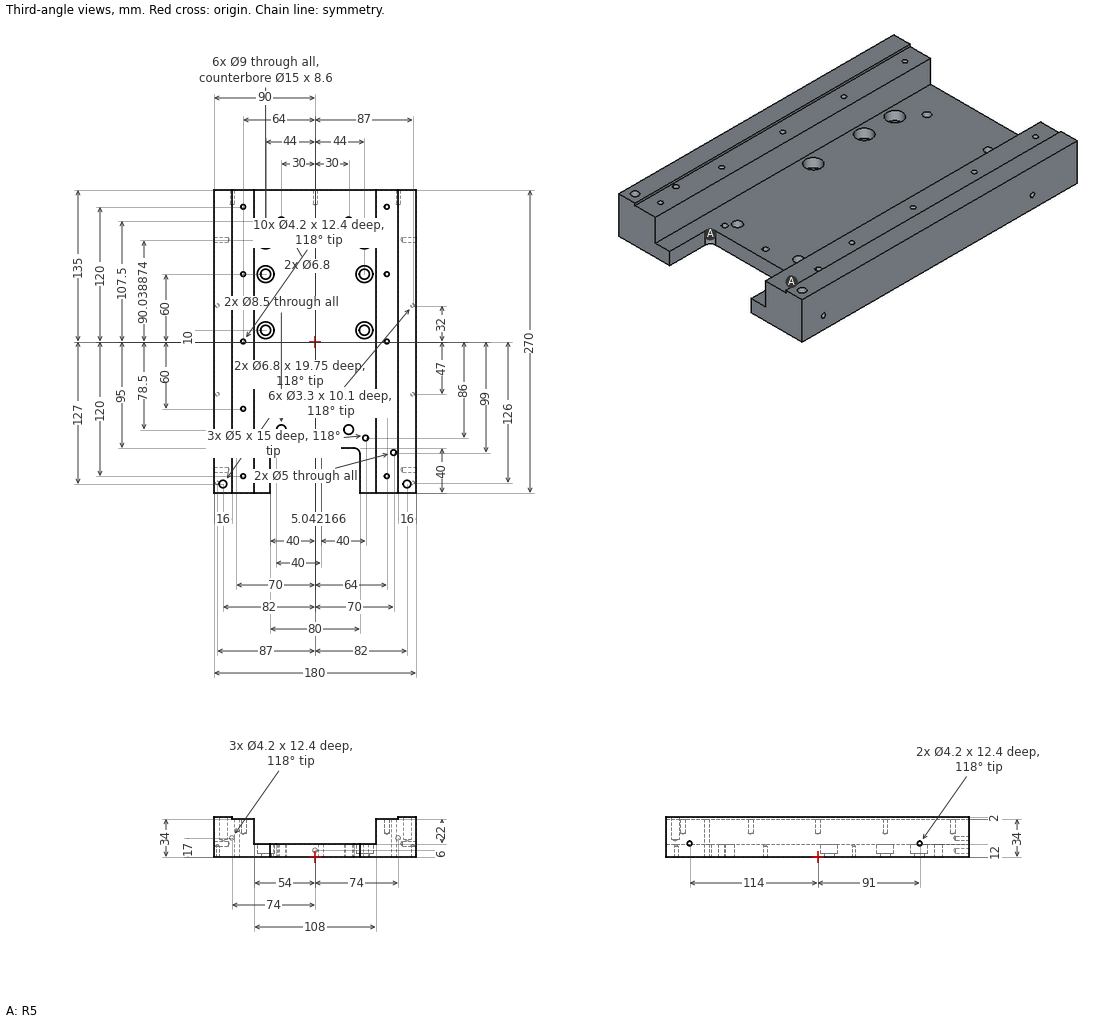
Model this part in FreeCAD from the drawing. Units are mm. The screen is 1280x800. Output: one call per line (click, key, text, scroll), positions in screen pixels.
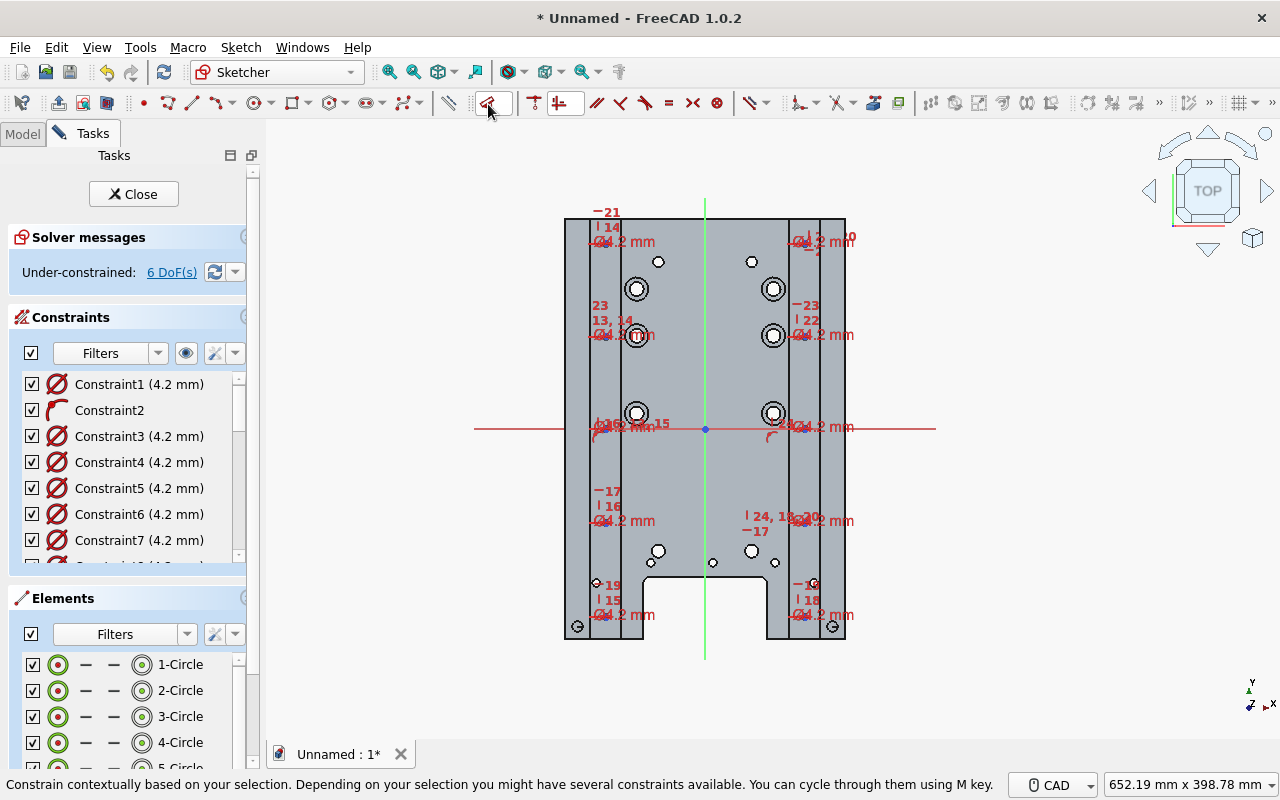
click(606, 429)
click(656, 463)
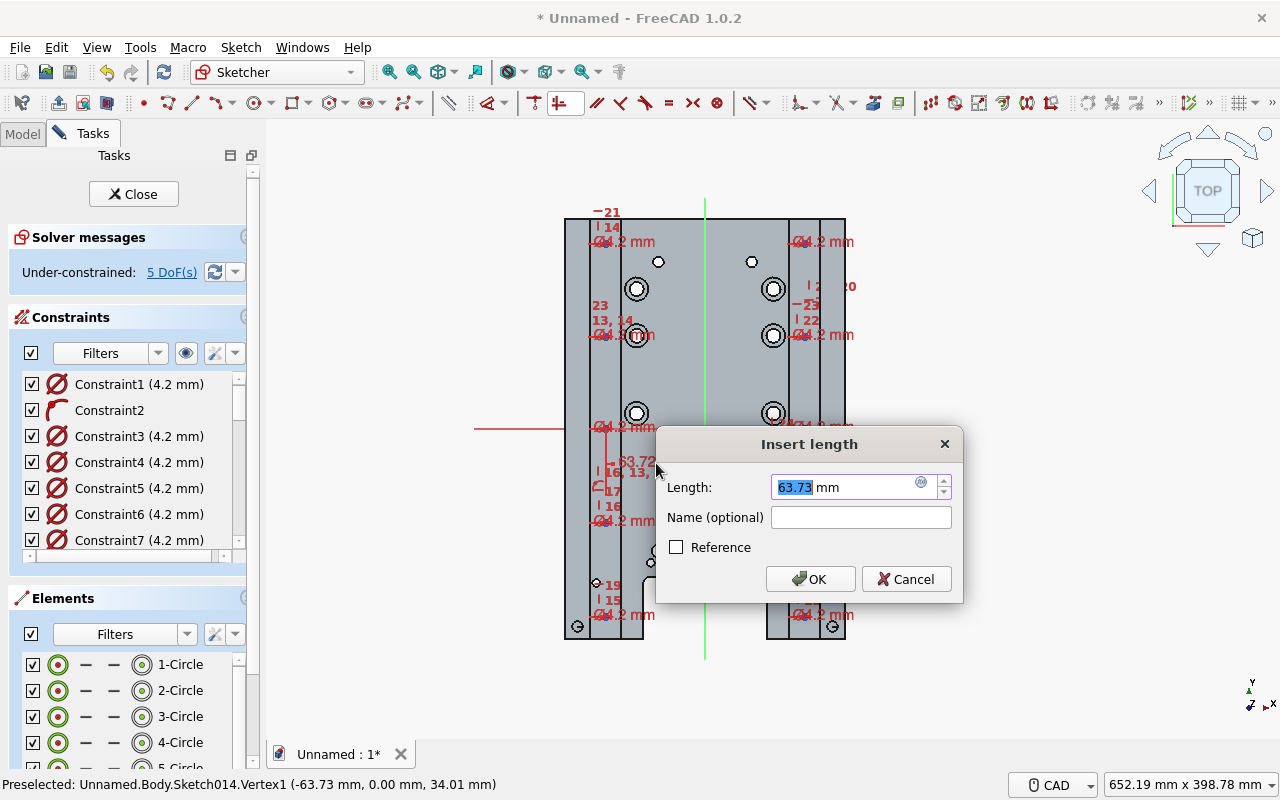
text(64)
key(Return)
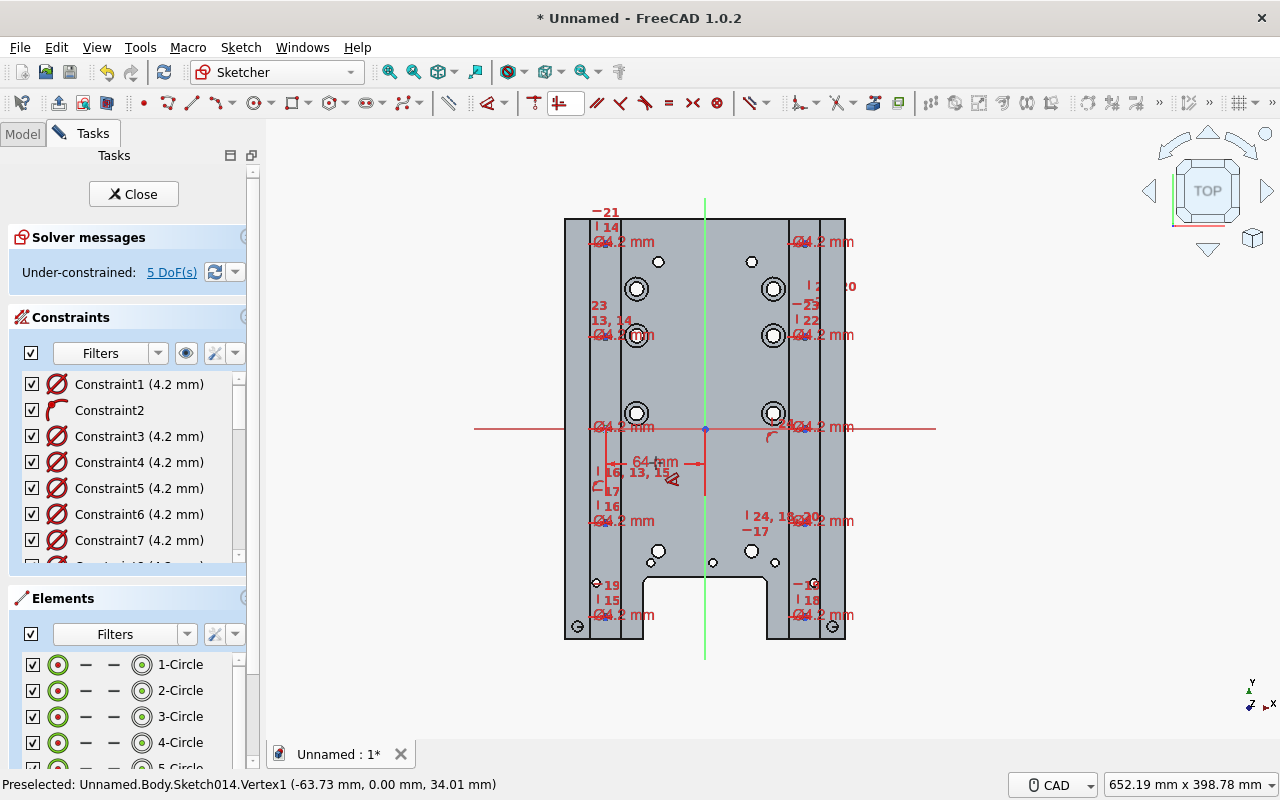
click(606, 337)
click(572, 383)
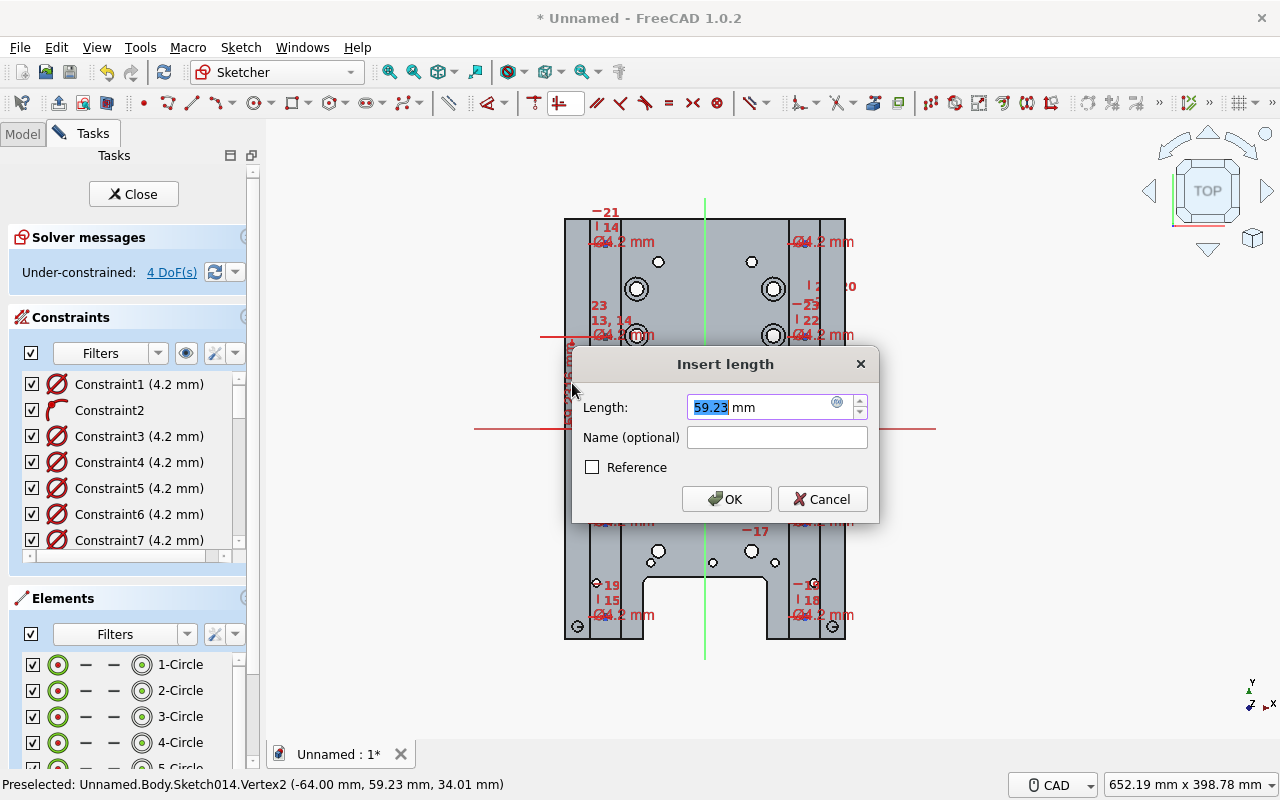
text(60)
key(Return)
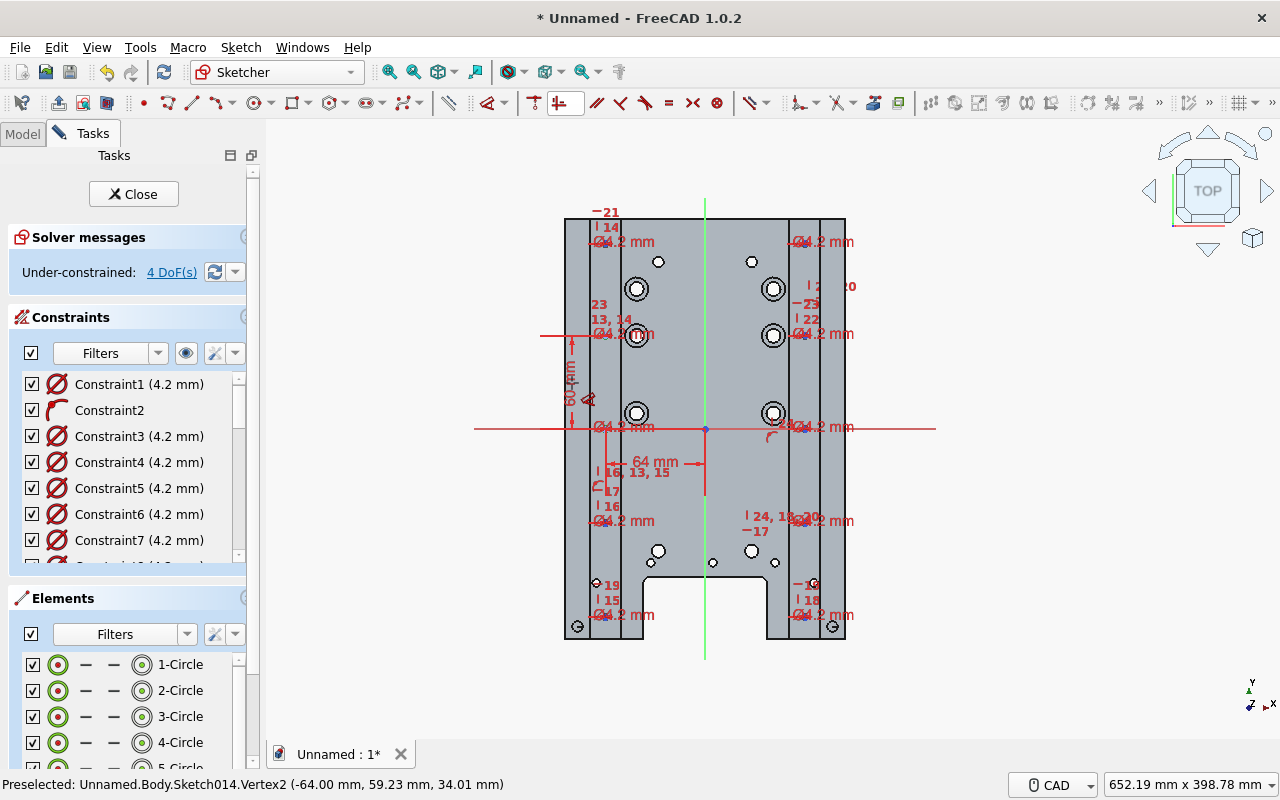
click(606, 523)
click(572, 476)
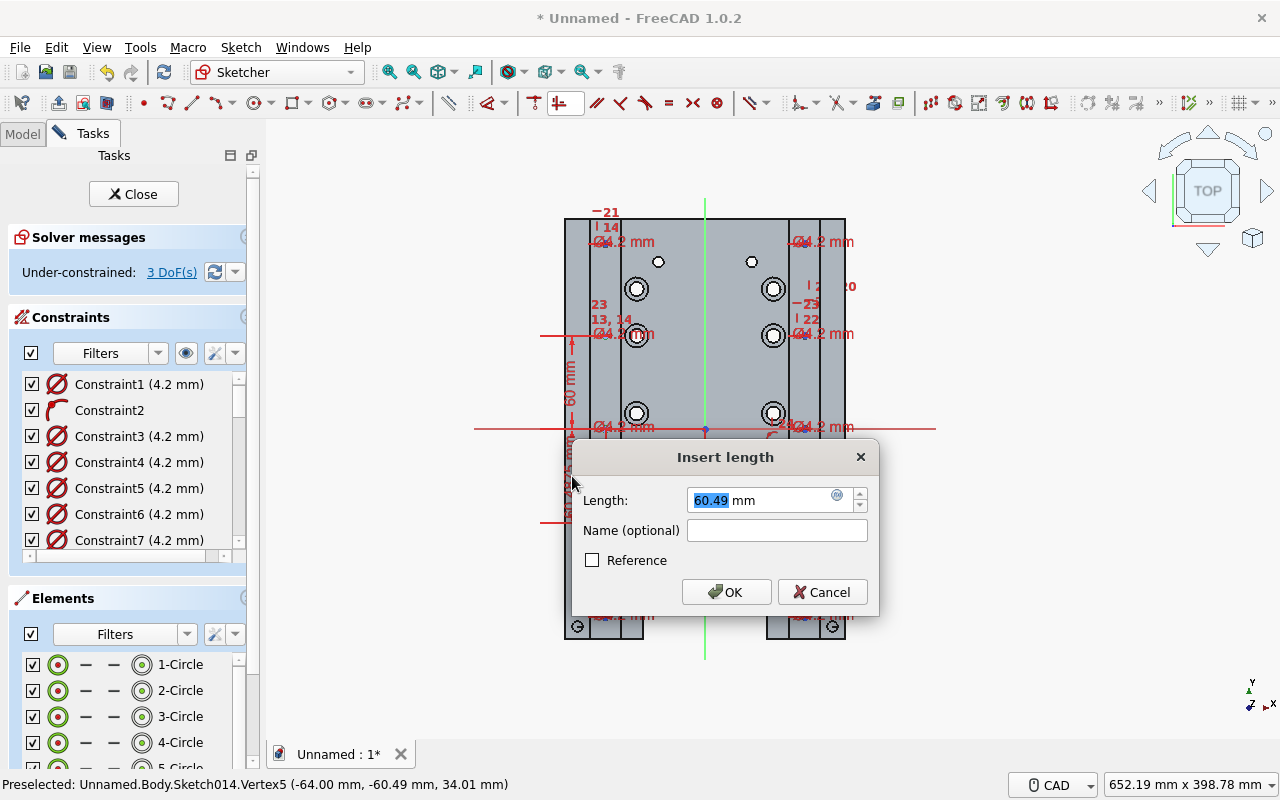
text(60)
key(Return)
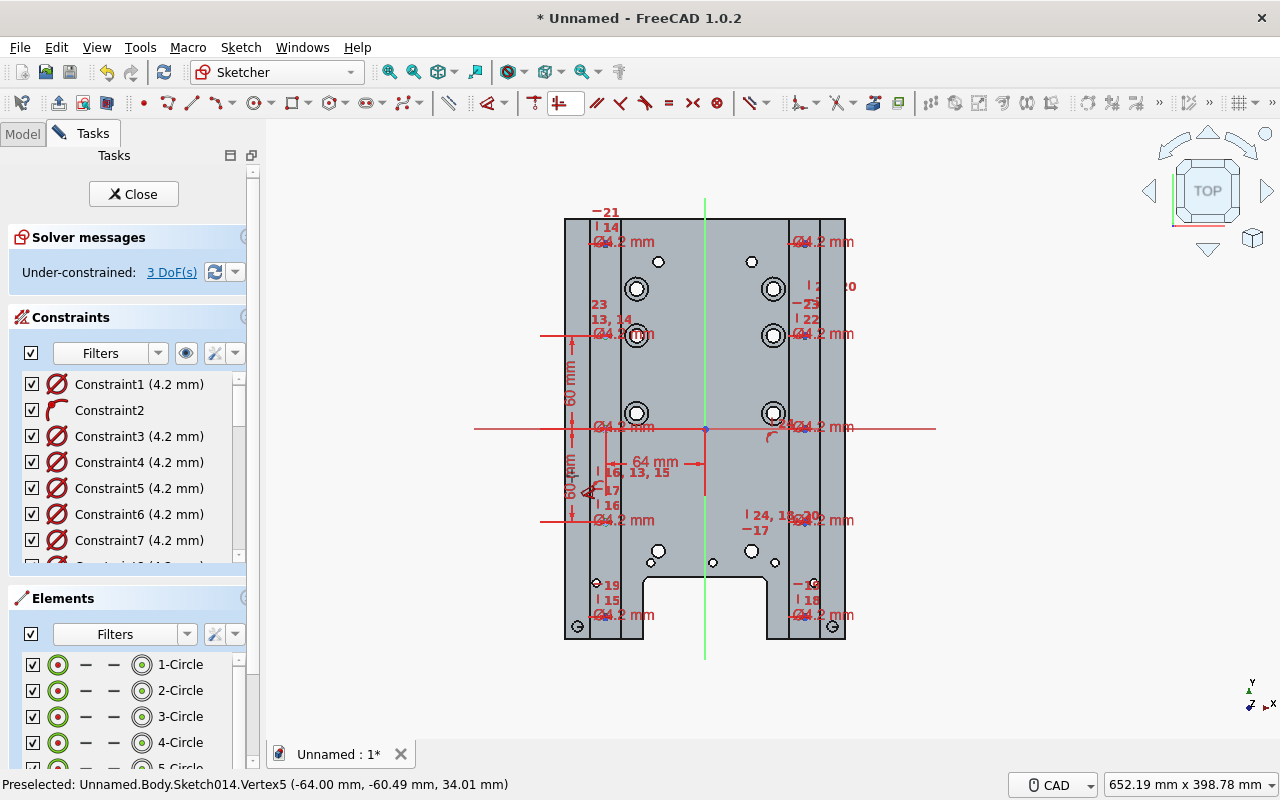
click(805, 522)
click(755, 556)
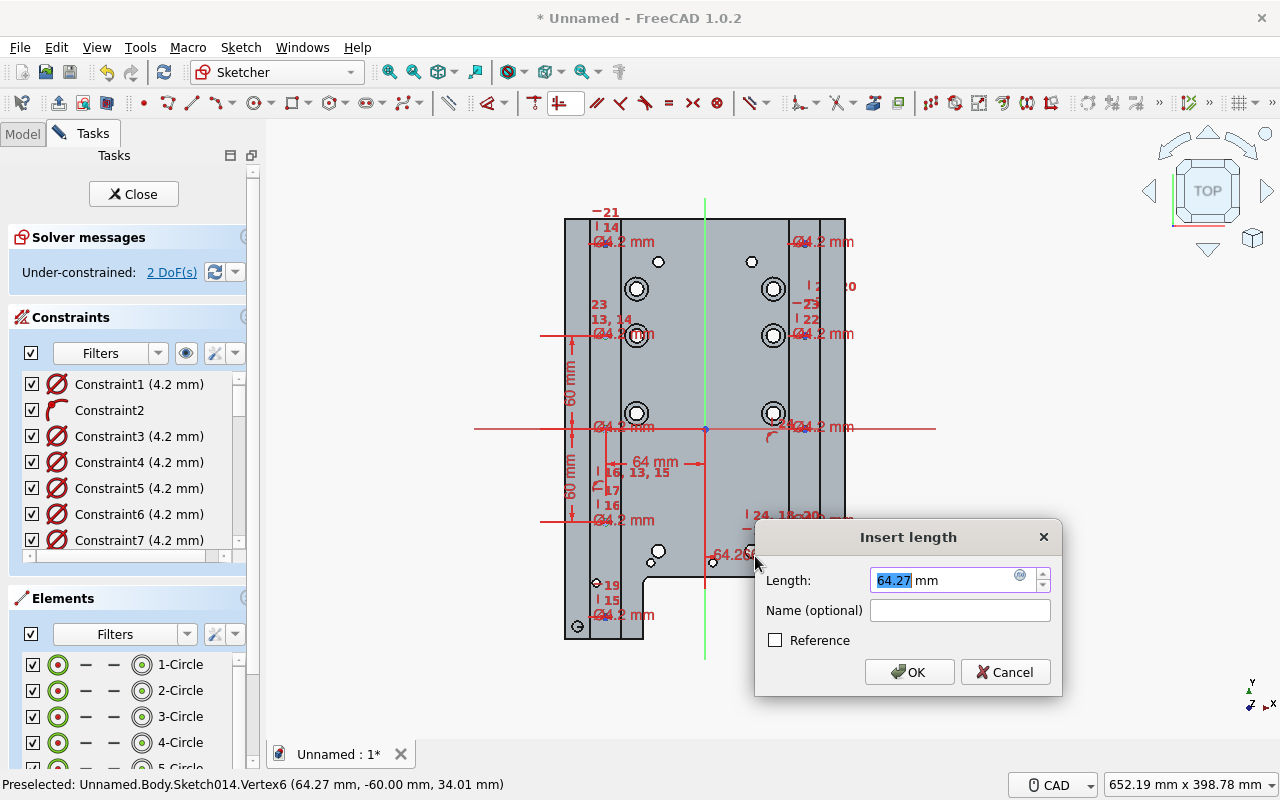
text(64)
key(Return)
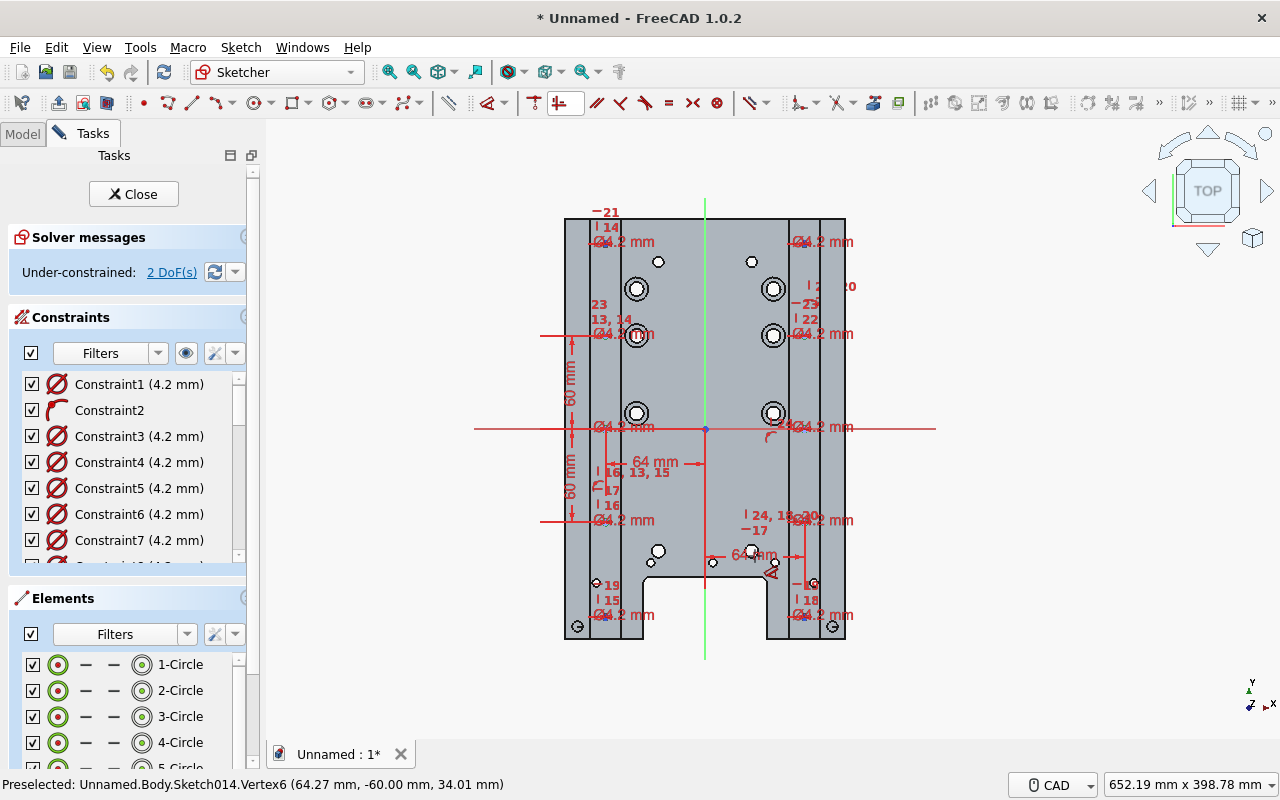
click(606, 244)
click(572, 337)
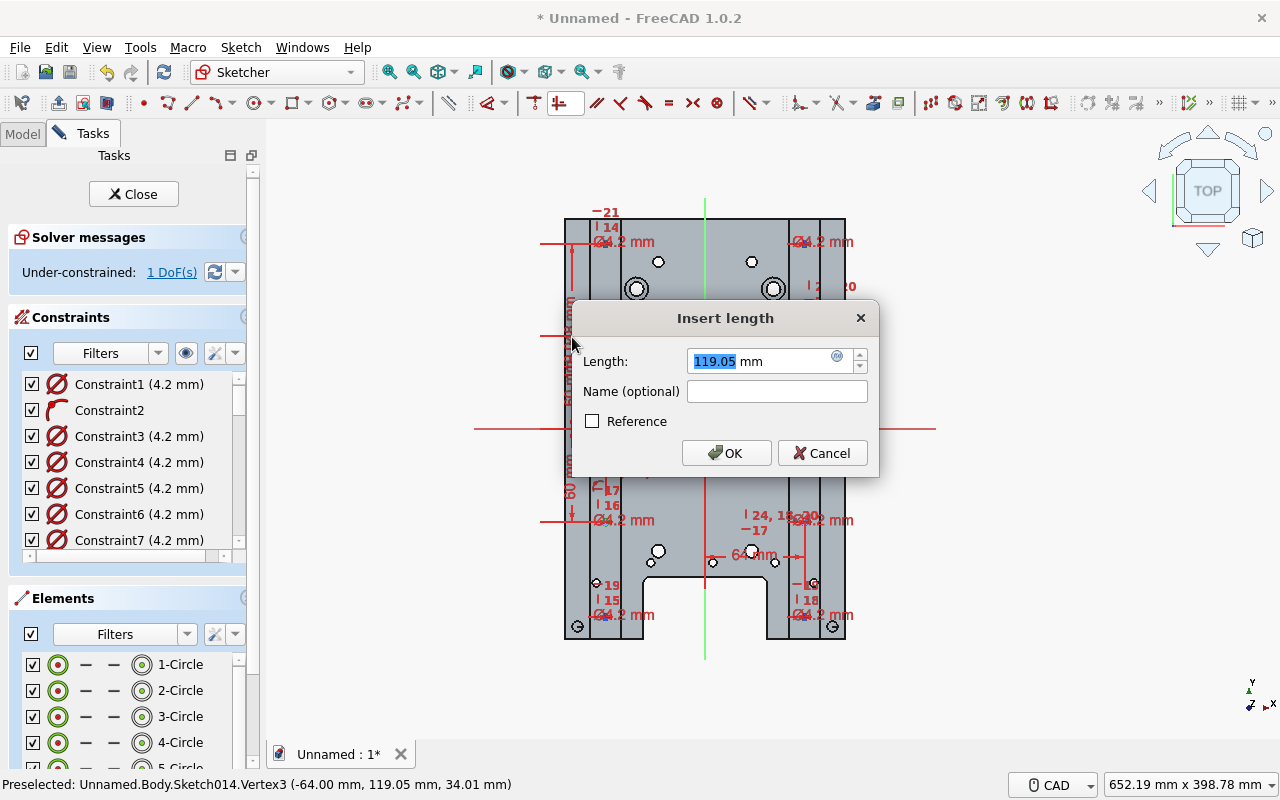
text(120)
key(Return)